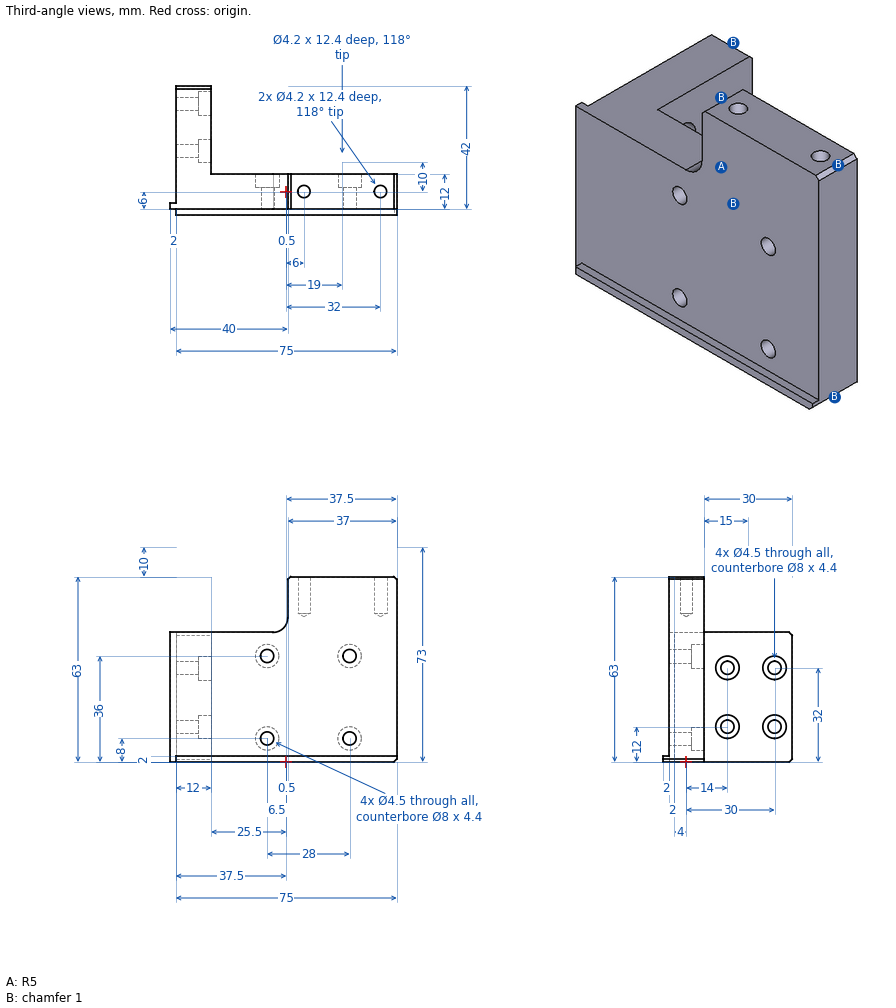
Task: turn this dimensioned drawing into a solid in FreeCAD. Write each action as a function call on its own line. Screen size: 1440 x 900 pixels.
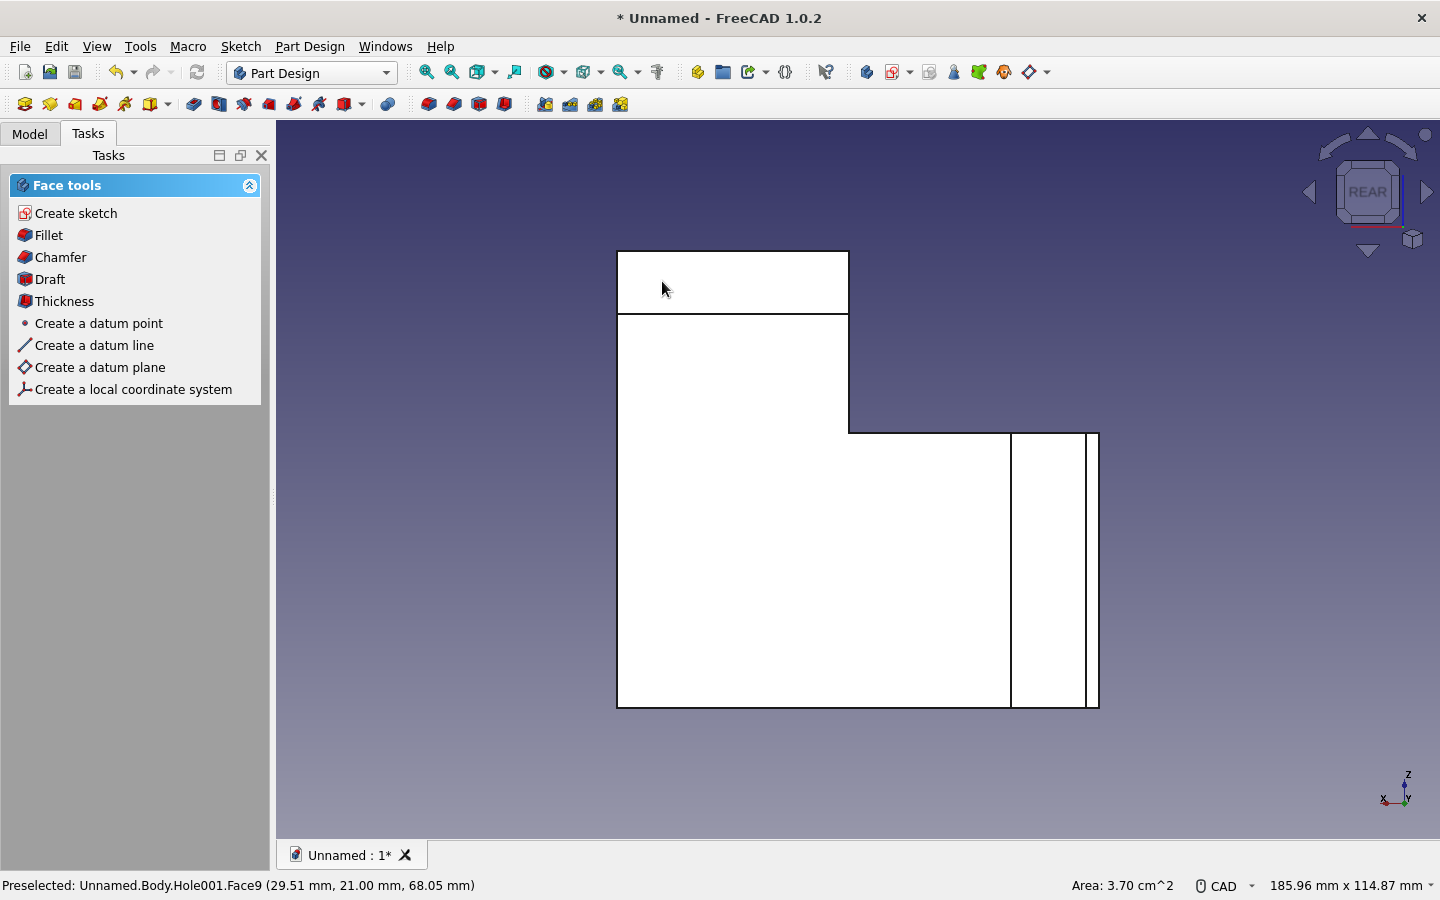
click(892, 72)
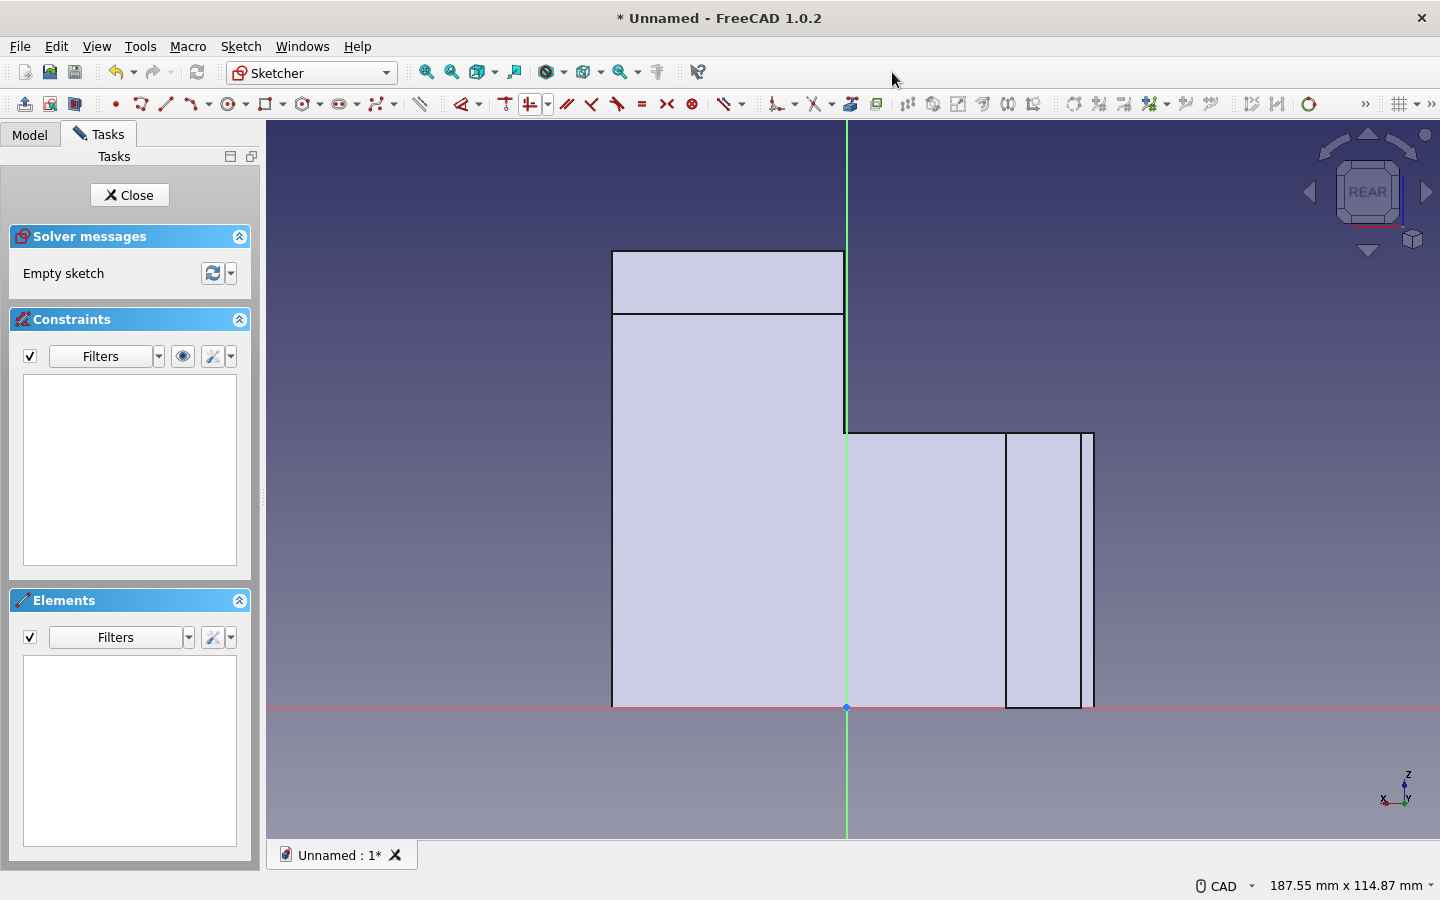
click(75, 104)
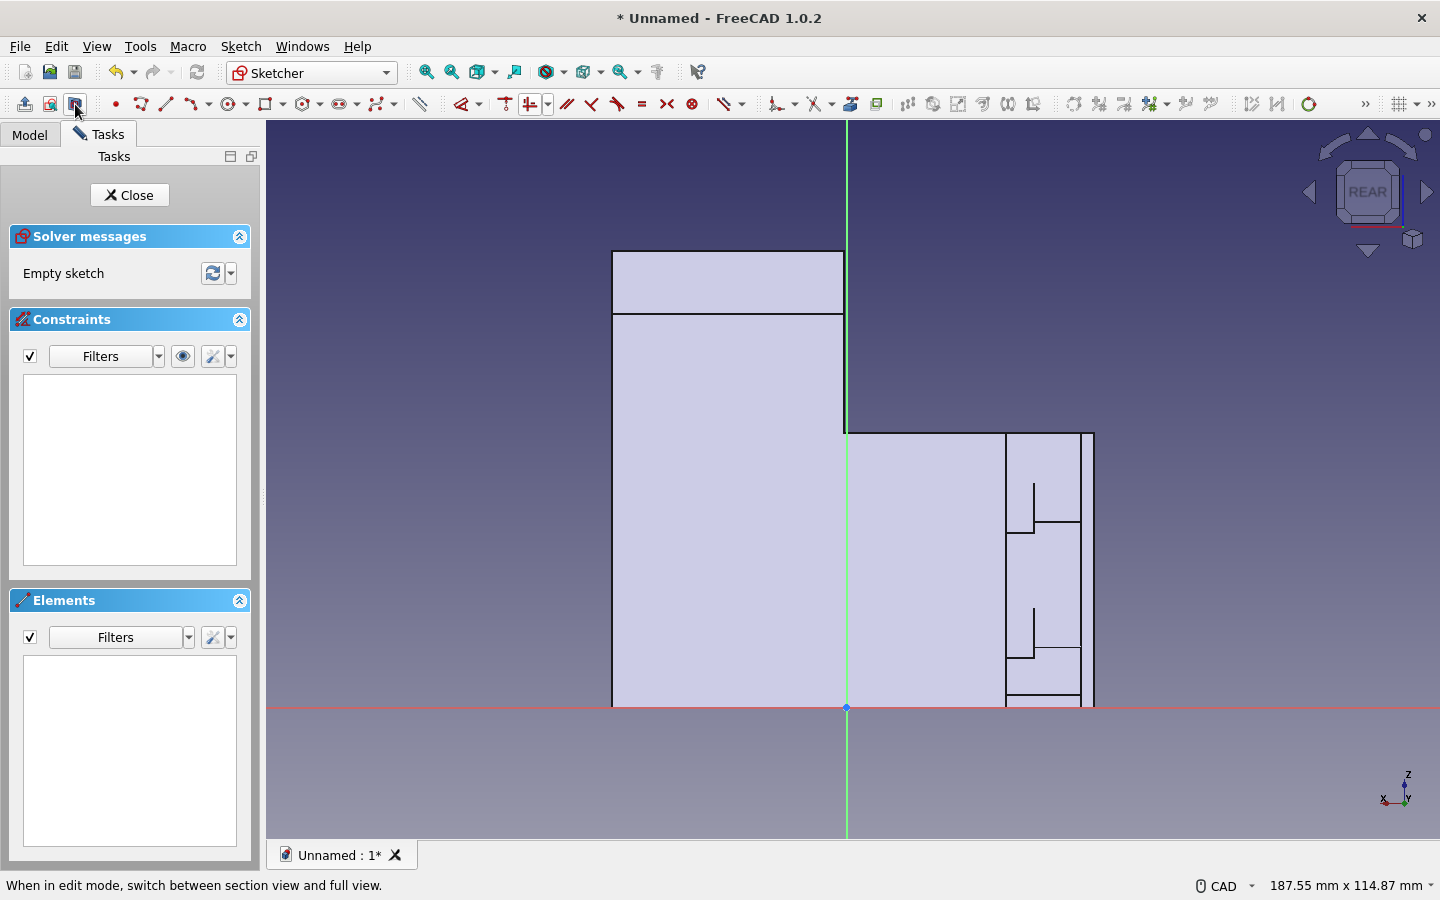
click(264, 104)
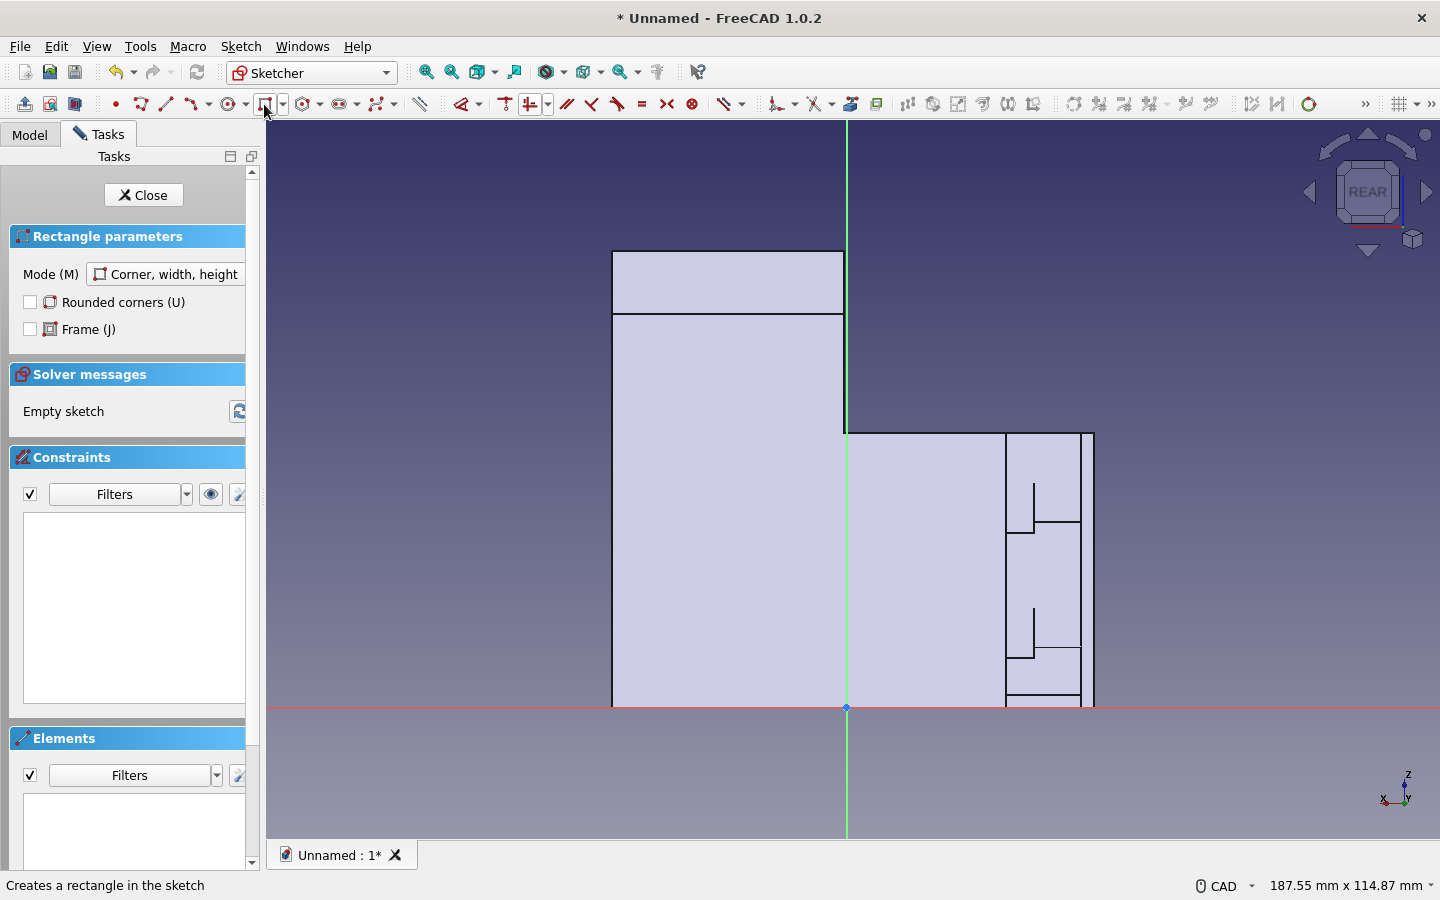
click(612, 251)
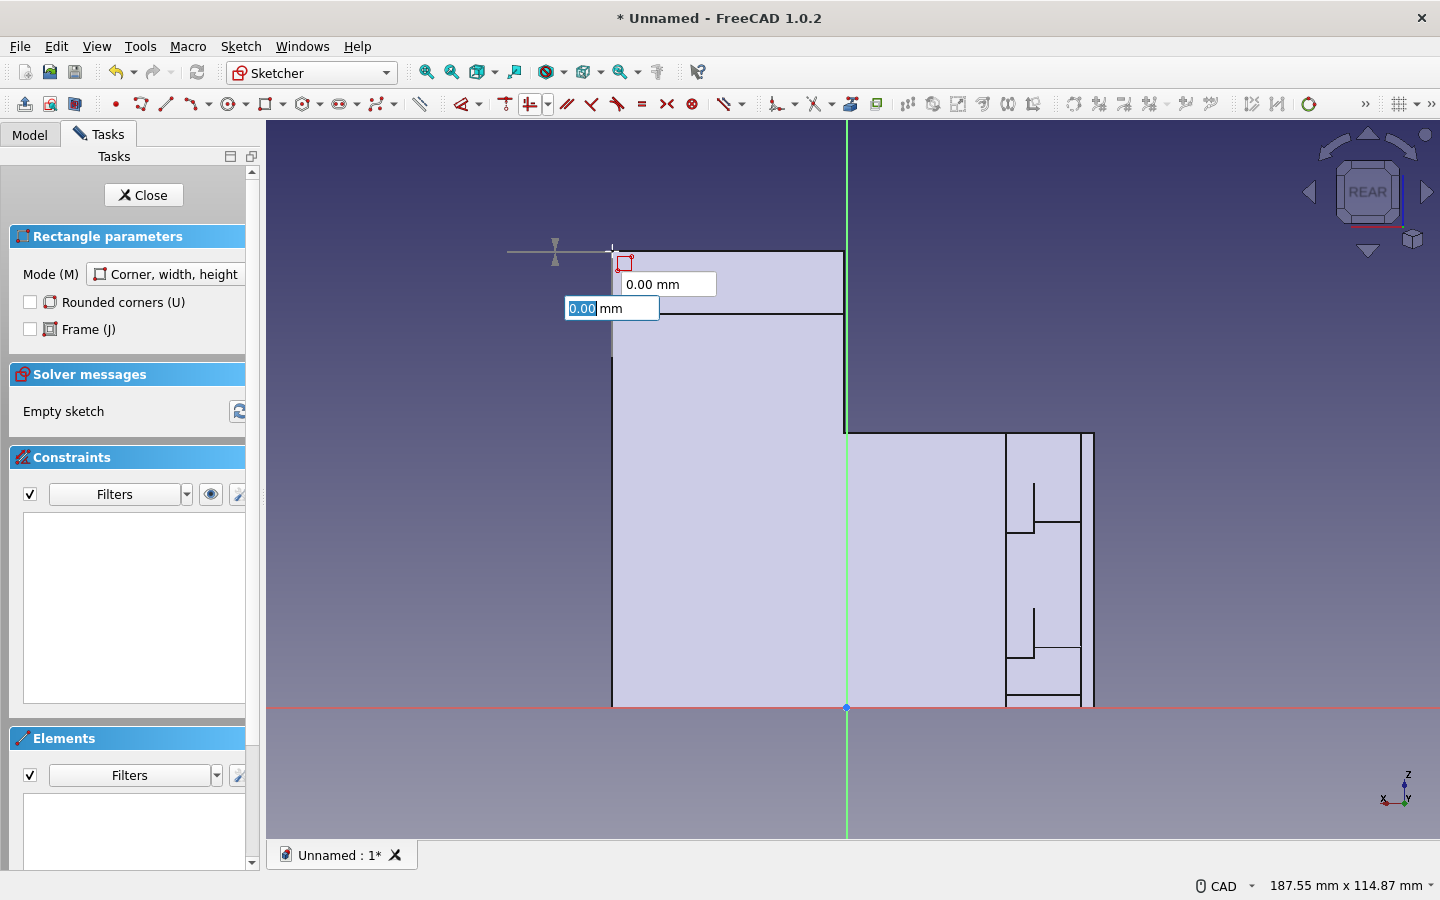
scroll(844, 314, up, 9)
move(839, 310)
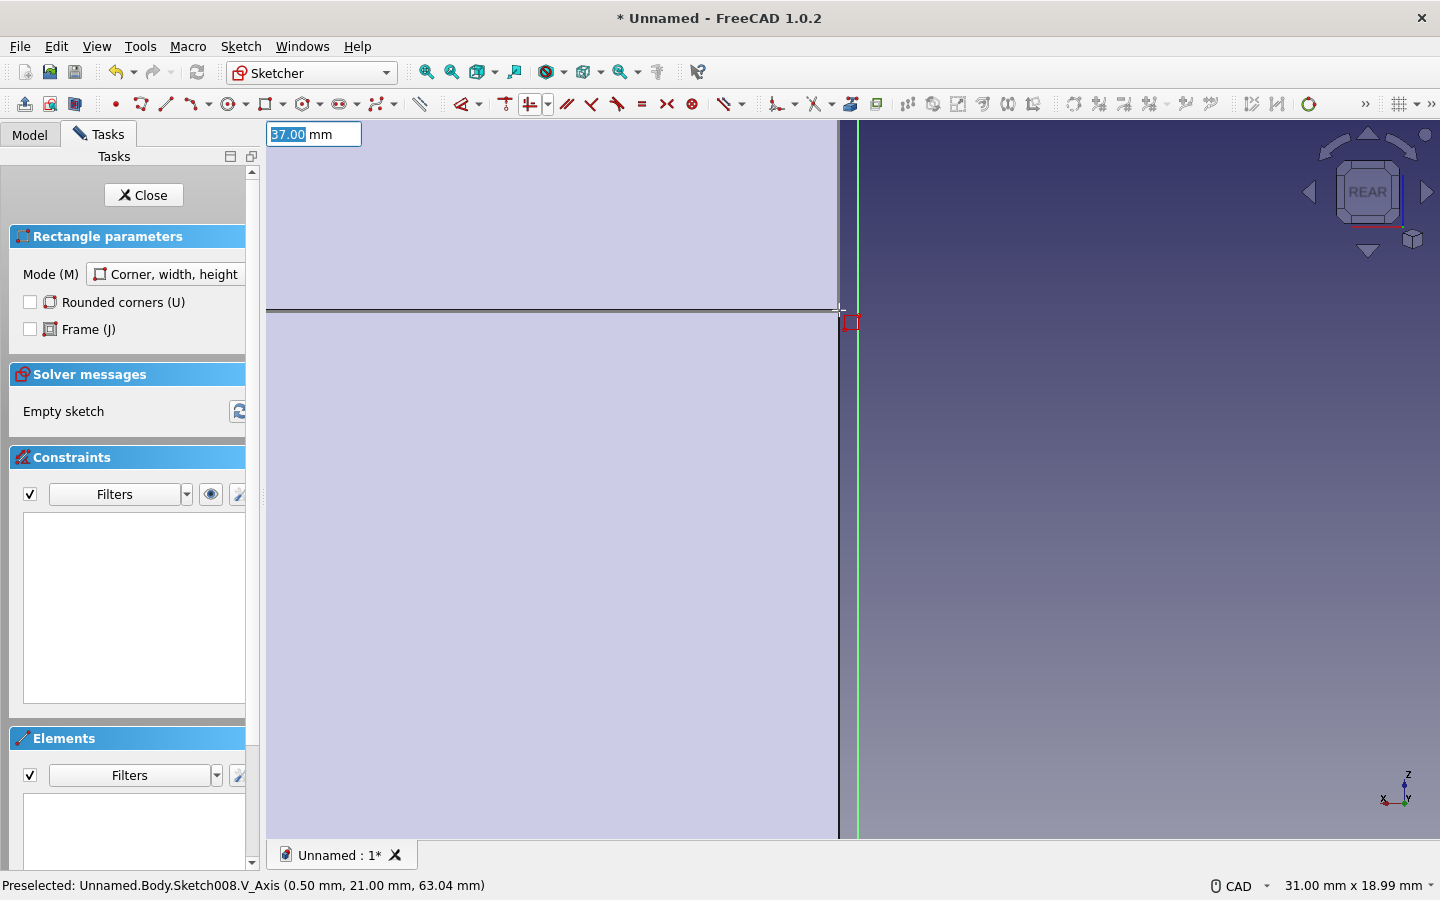
text(37)
key(Tab)
text(10)
key(Return)
key(Escape)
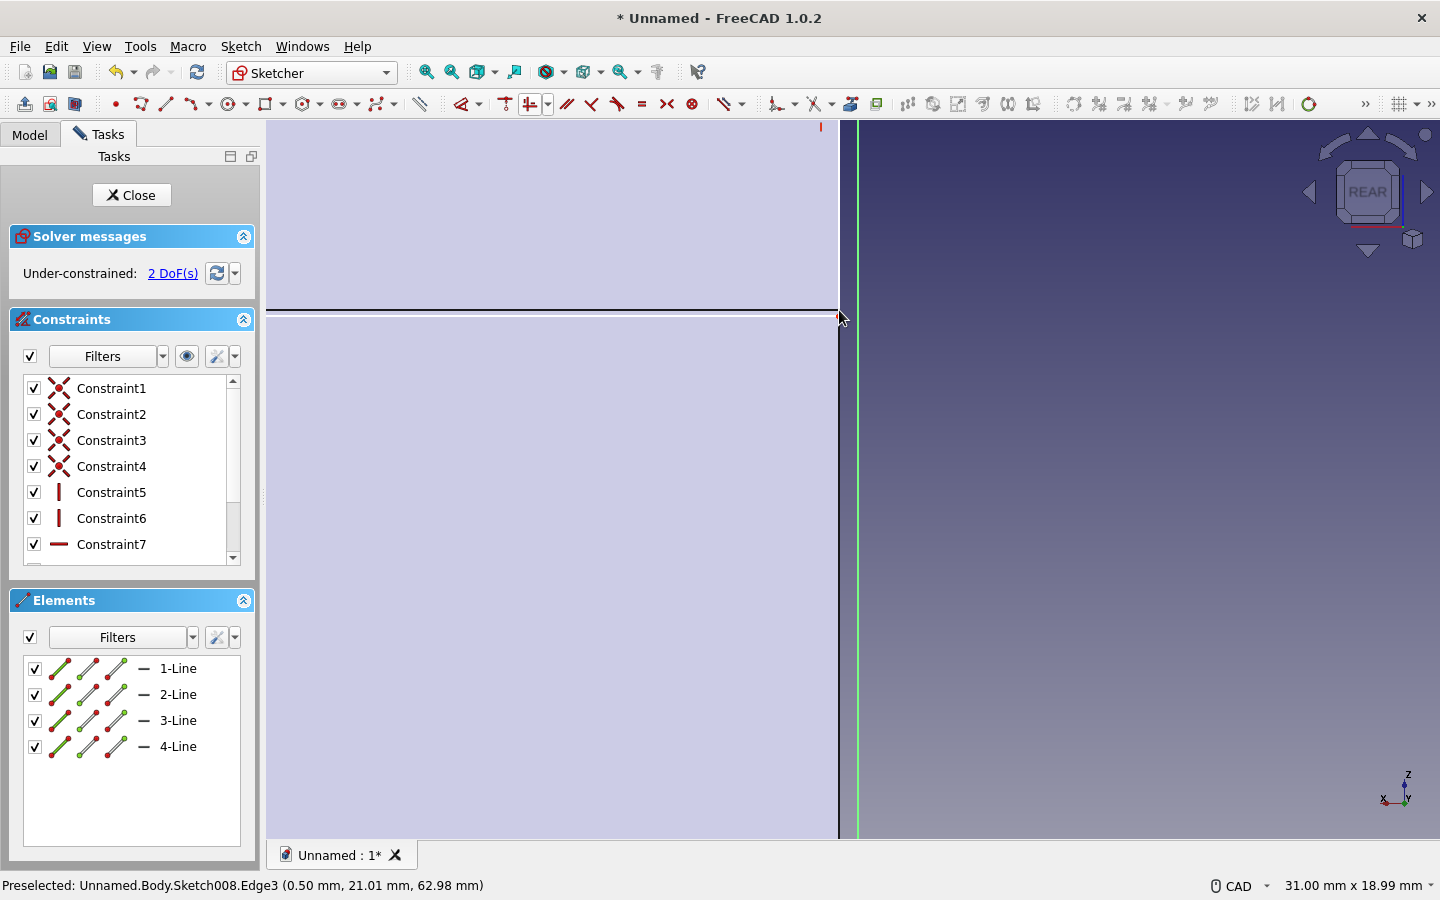
click(460, 104)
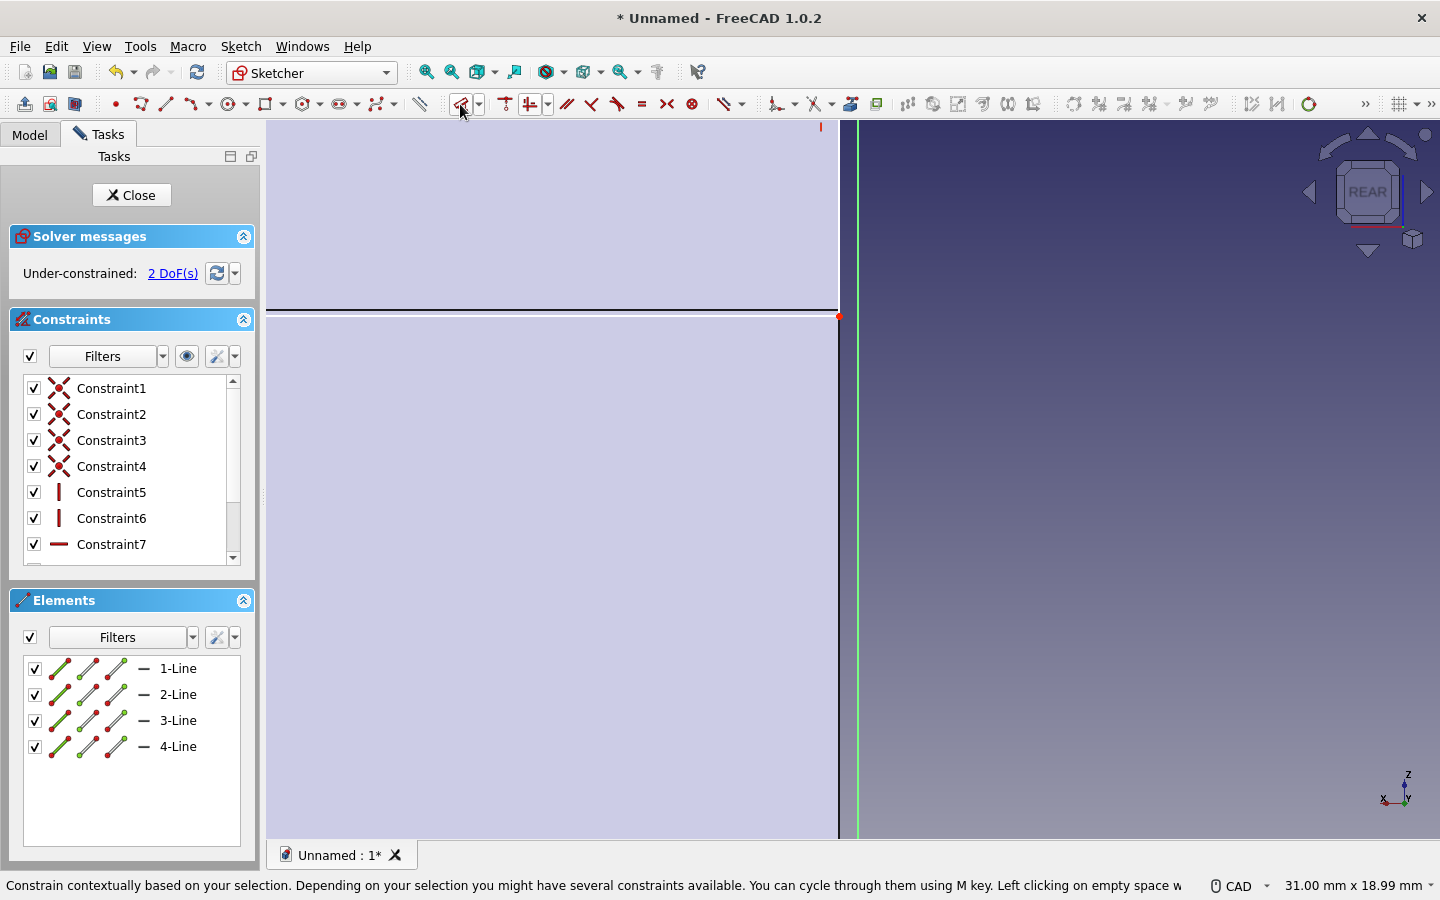
scroll(911, 314, down, 9)